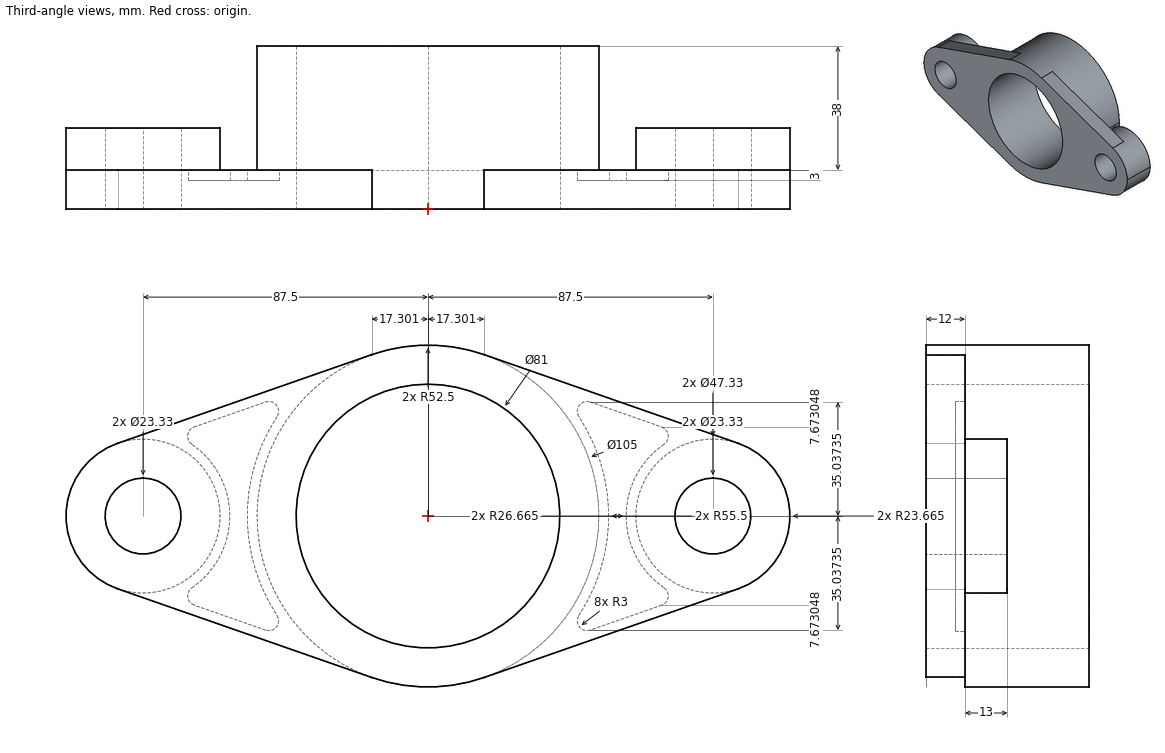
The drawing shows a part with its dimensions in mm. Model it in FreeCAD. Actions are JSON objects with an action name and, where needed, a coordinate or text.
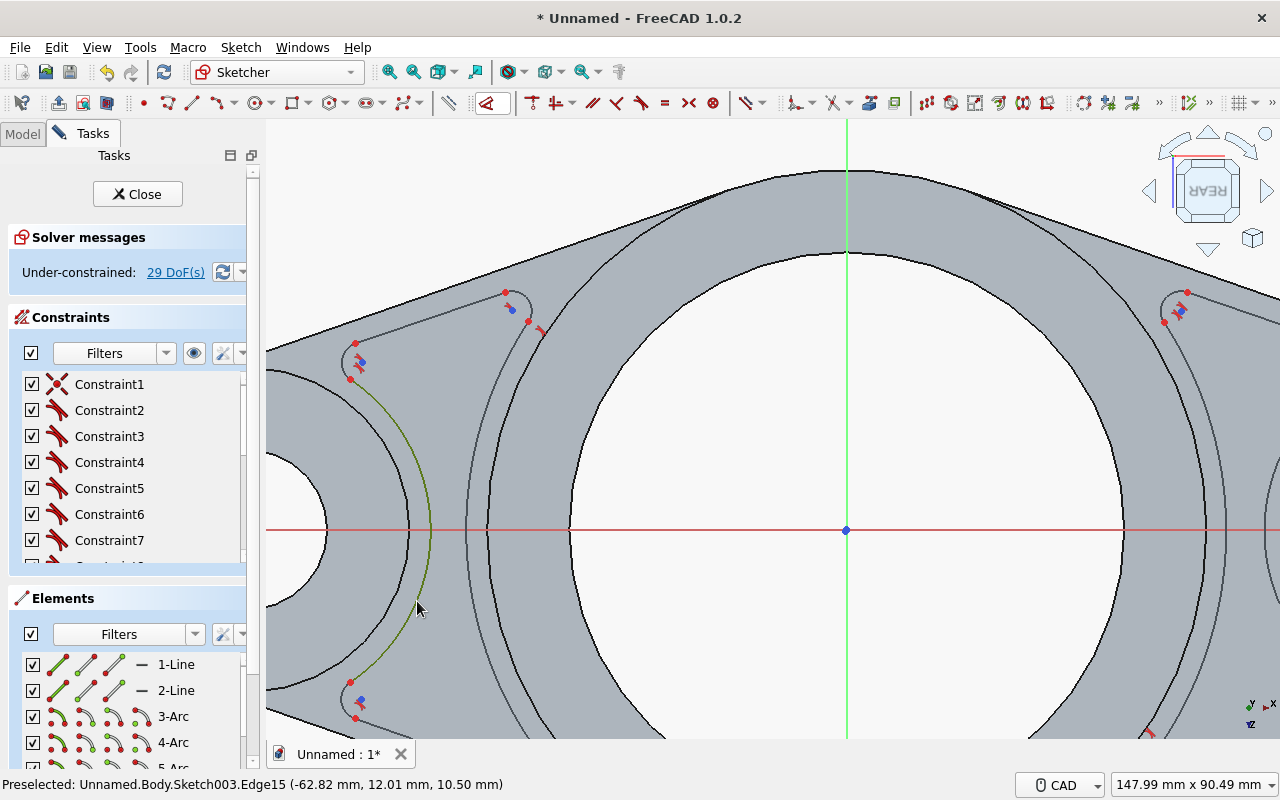
{"action": "left_click", "coordinate": [342, 693]}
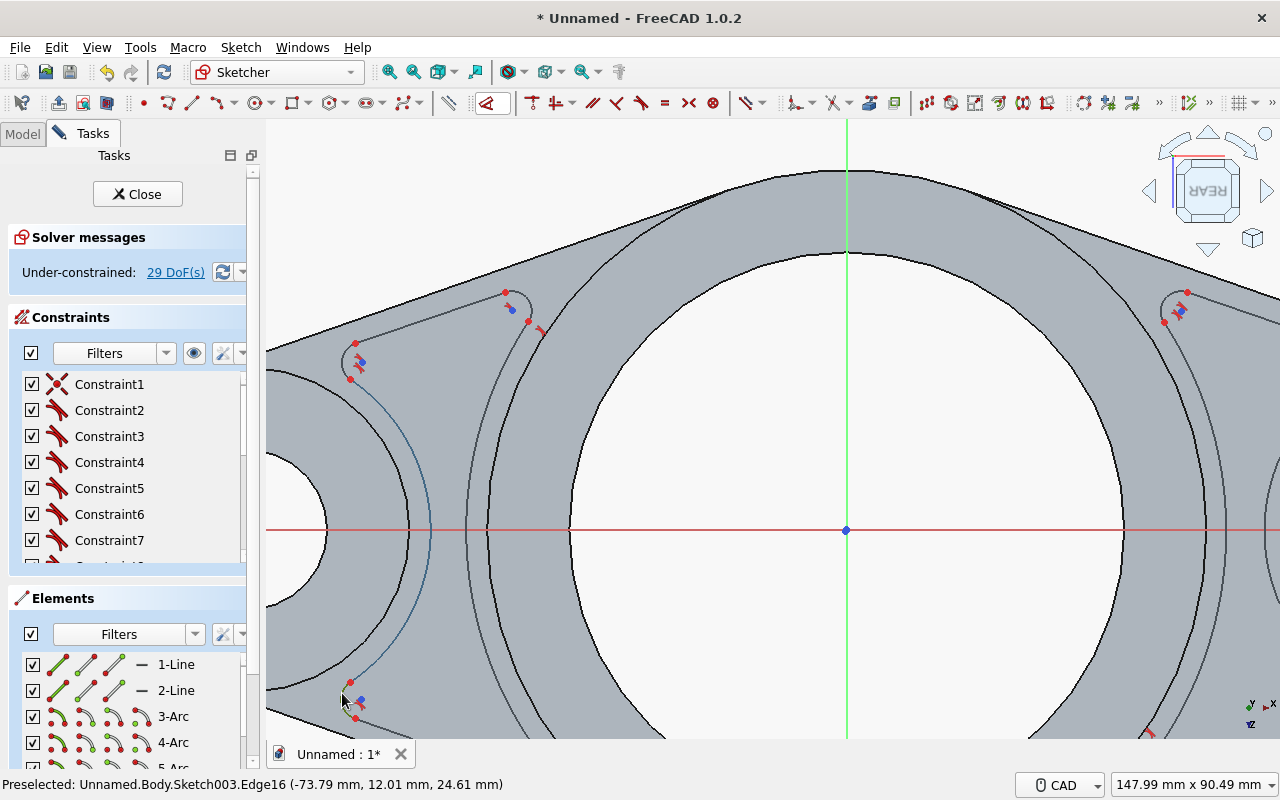
{"action": "left_click", "coordinate": [642, 104]}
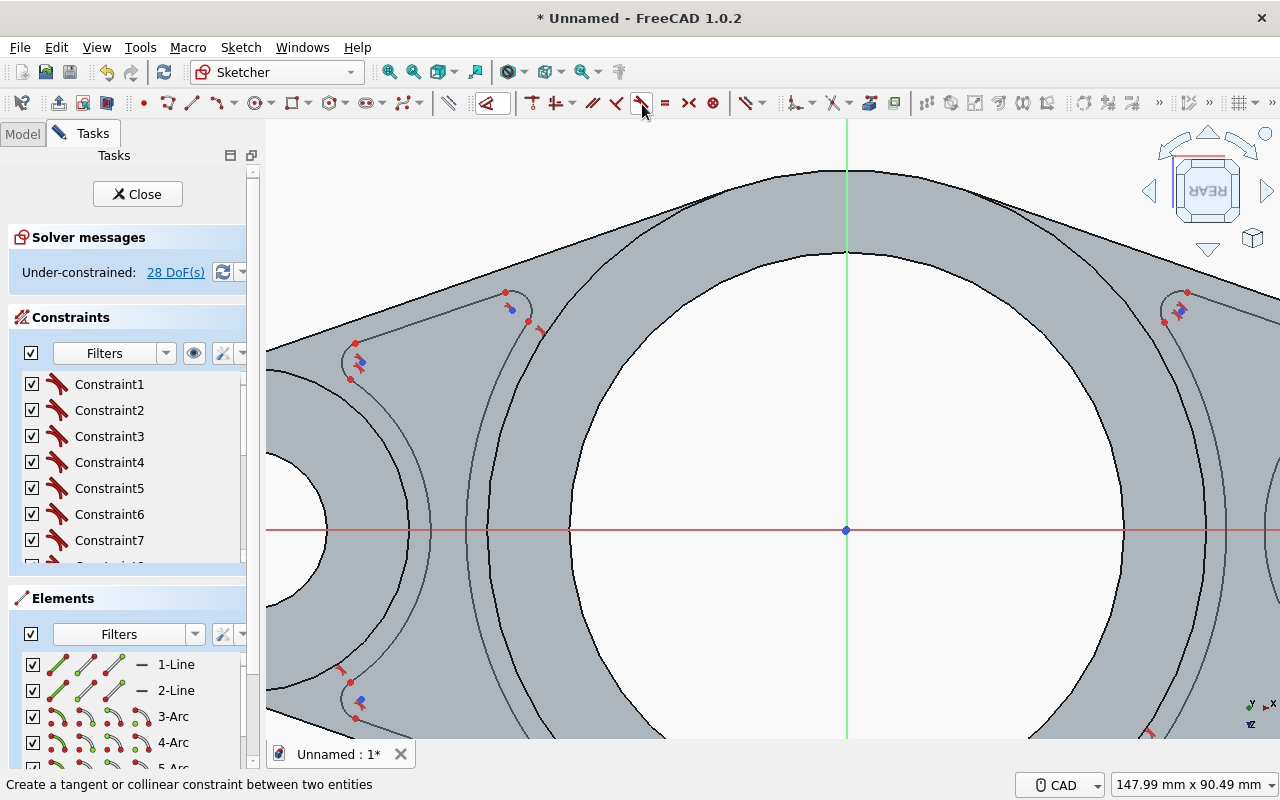
{"action": "scroll", "coordinate": [531, 306], "scroll_direction": "down", "scroll_amount": 3}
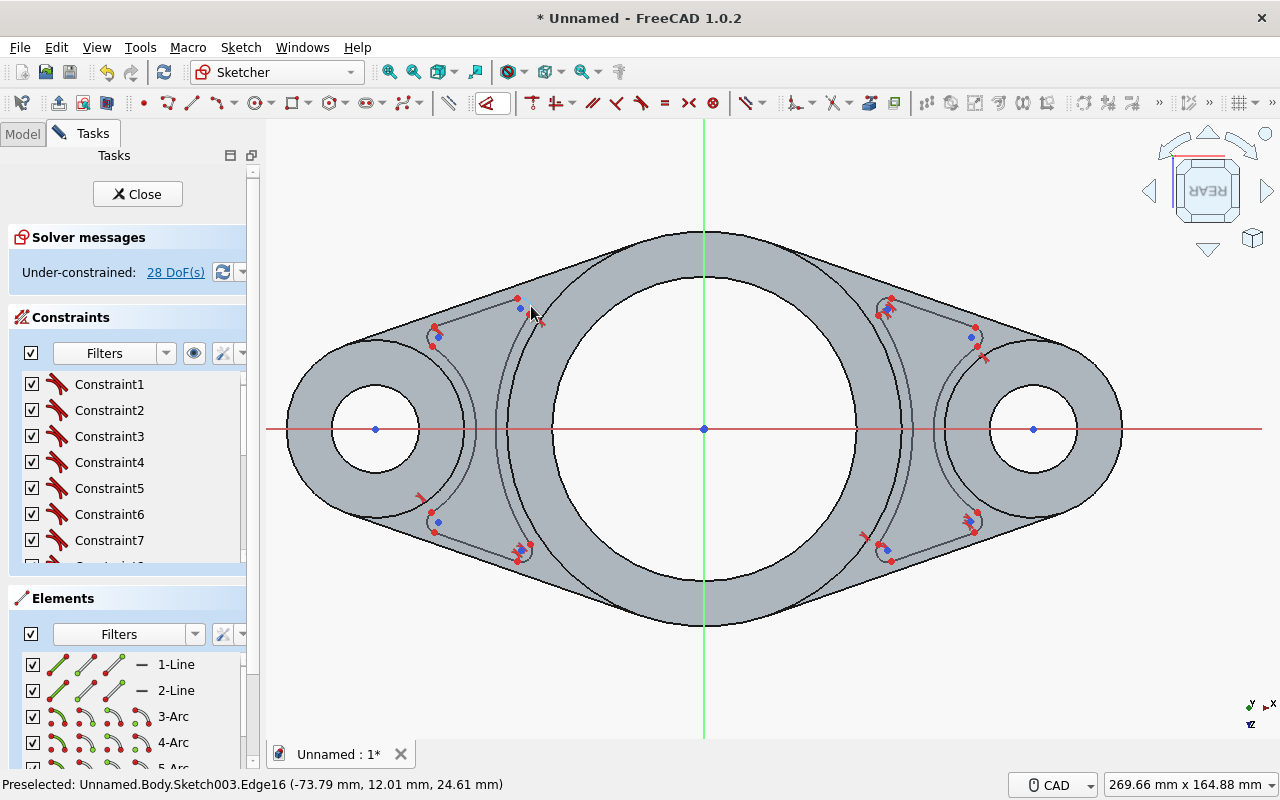
{"action": "left_click", "coordinate": [907, 478]}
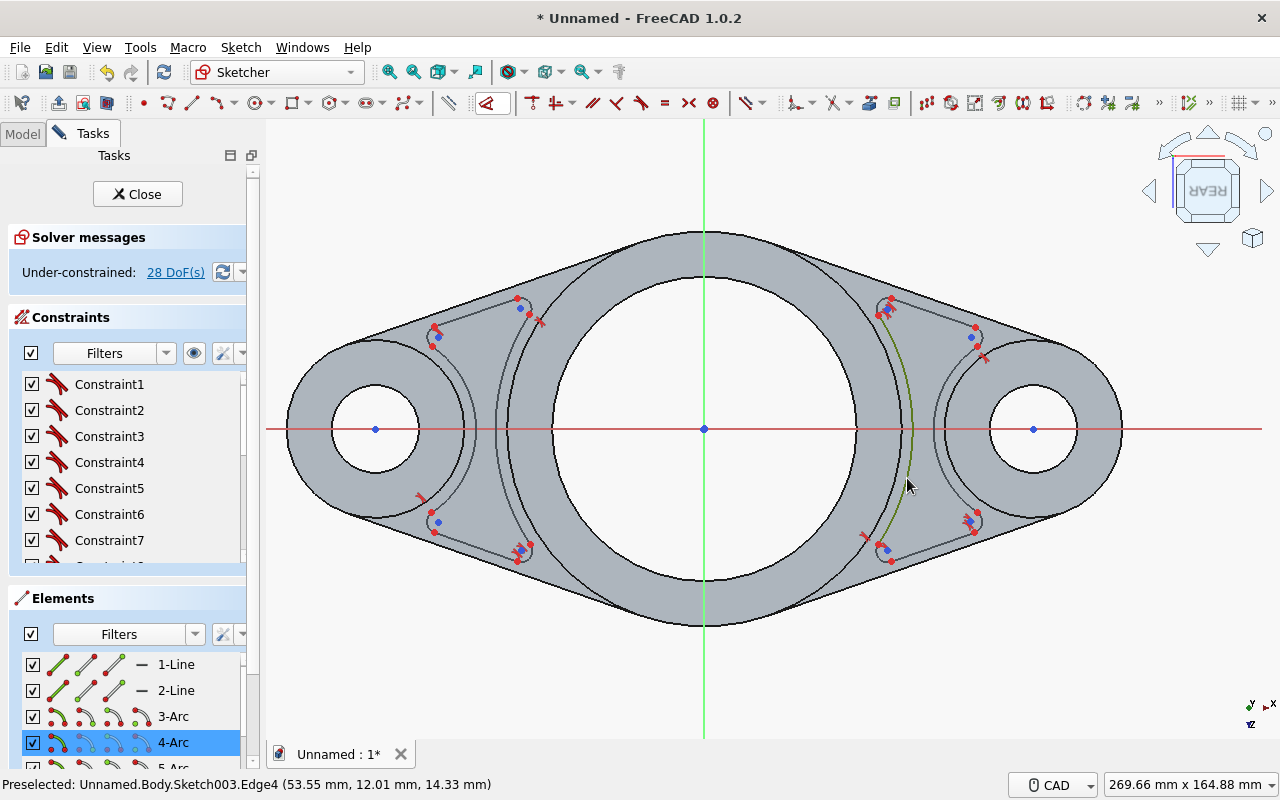
{"action": "left_click", "coordinate": [501, 381]}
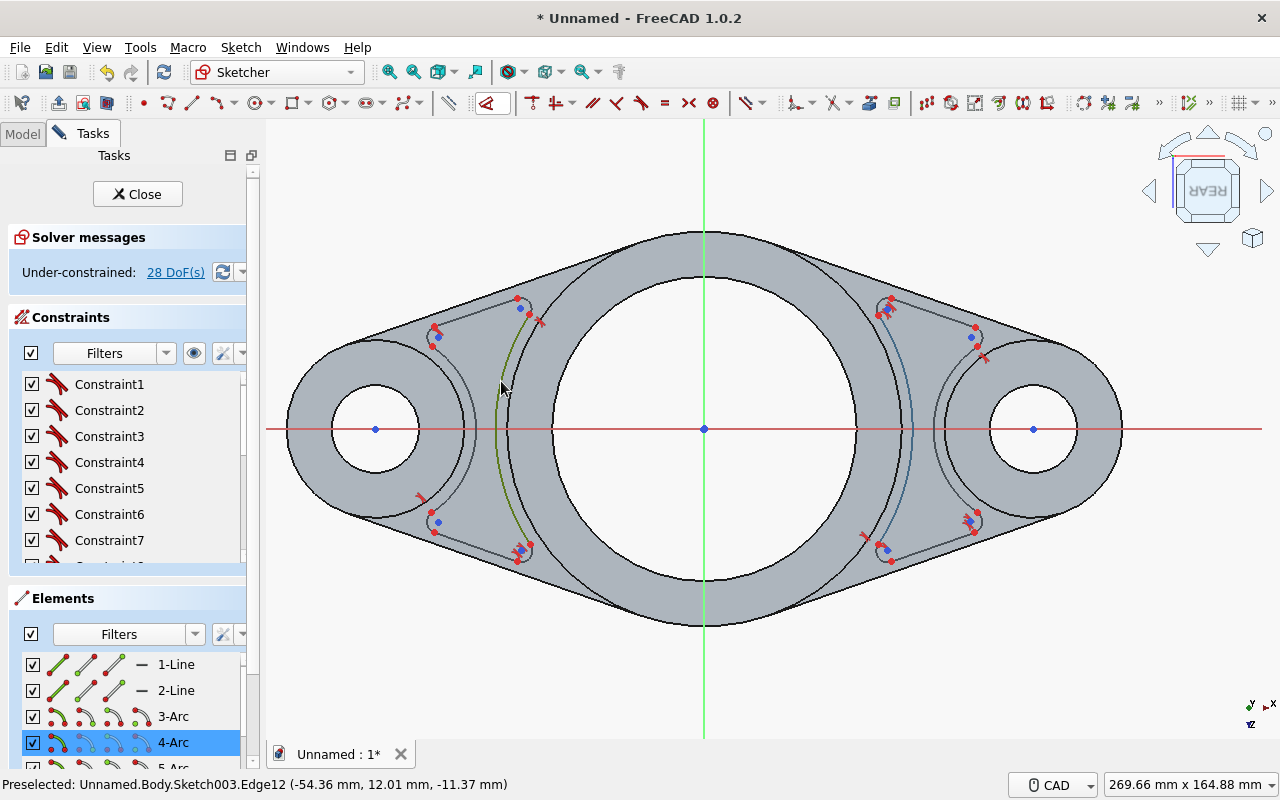
{"action": "left_click", "coordinate": [532, 104]}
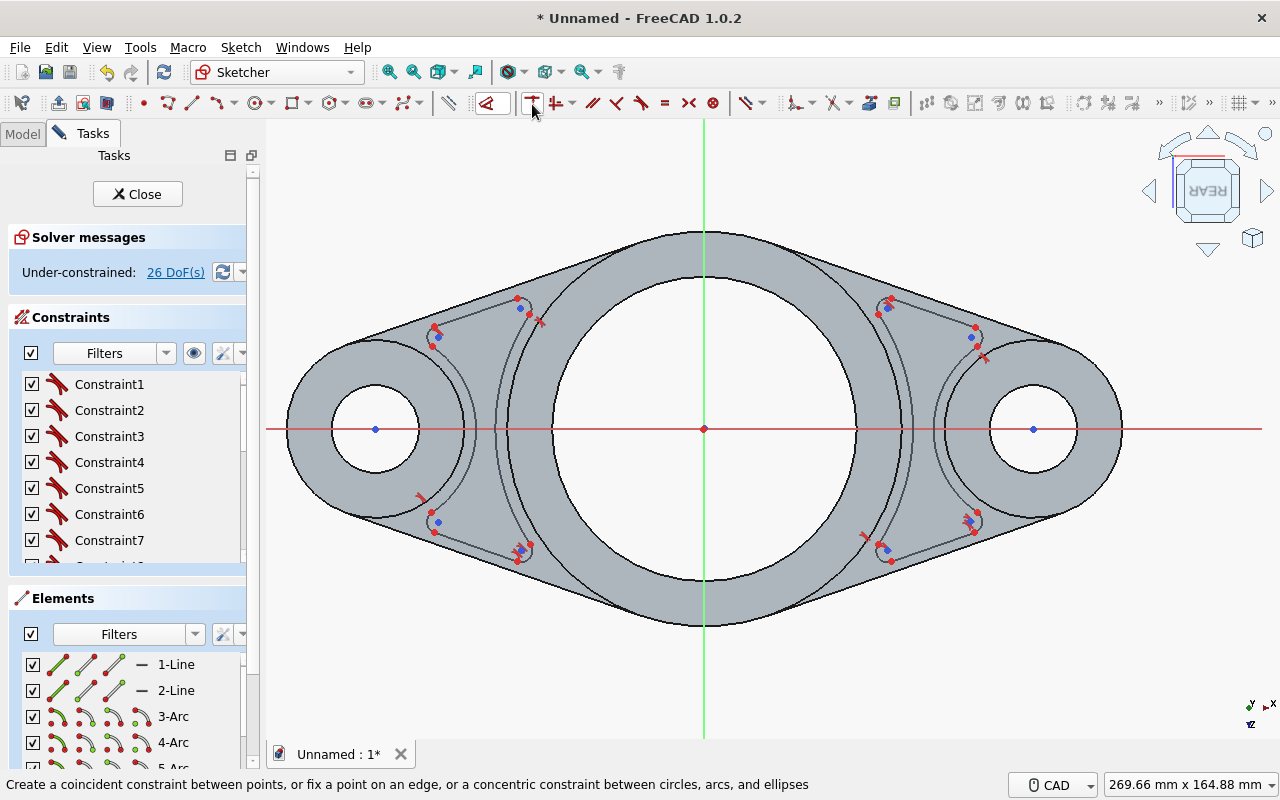
{"action": "scroll", "coordinate": [704, 429], "scroll_direction": "up", "scroll_amount": 7}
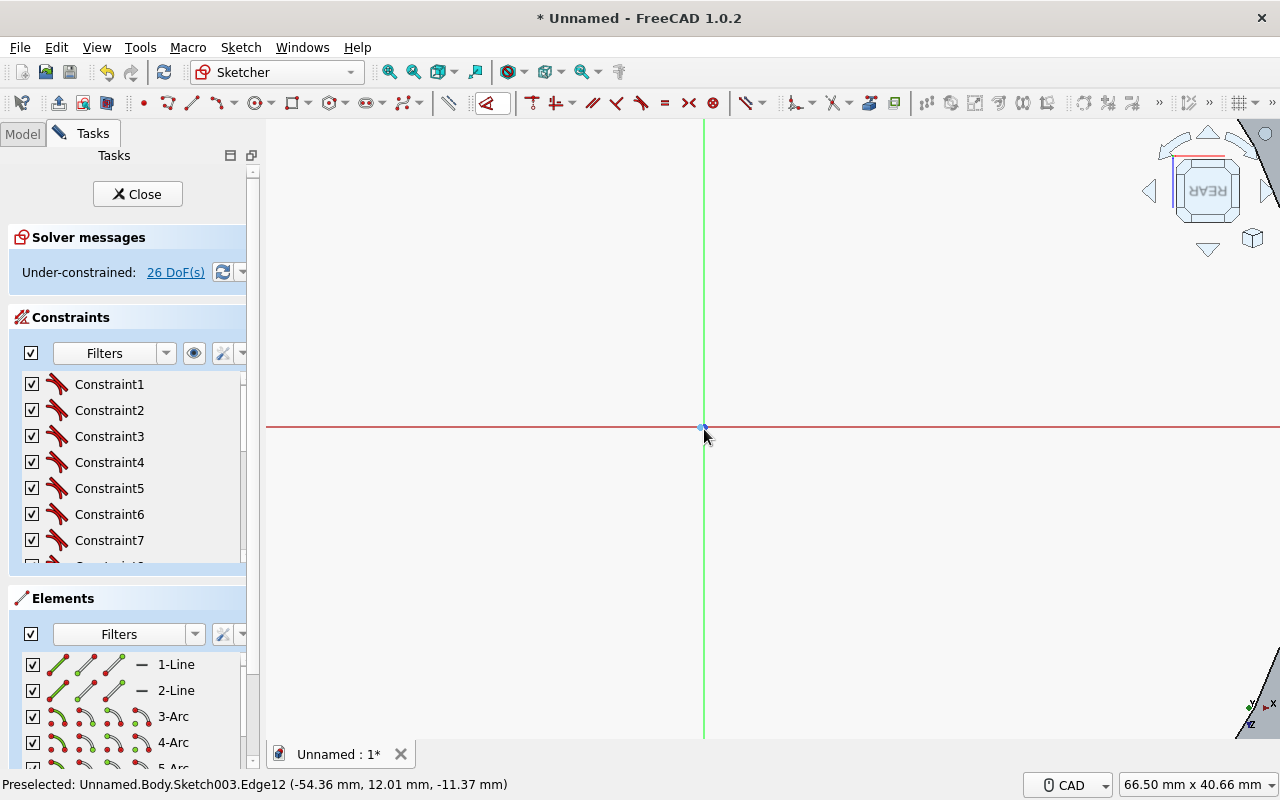
{"action": "left_click_drag", "start_coordinate": [691, 417], "coordinate": [714, 438]}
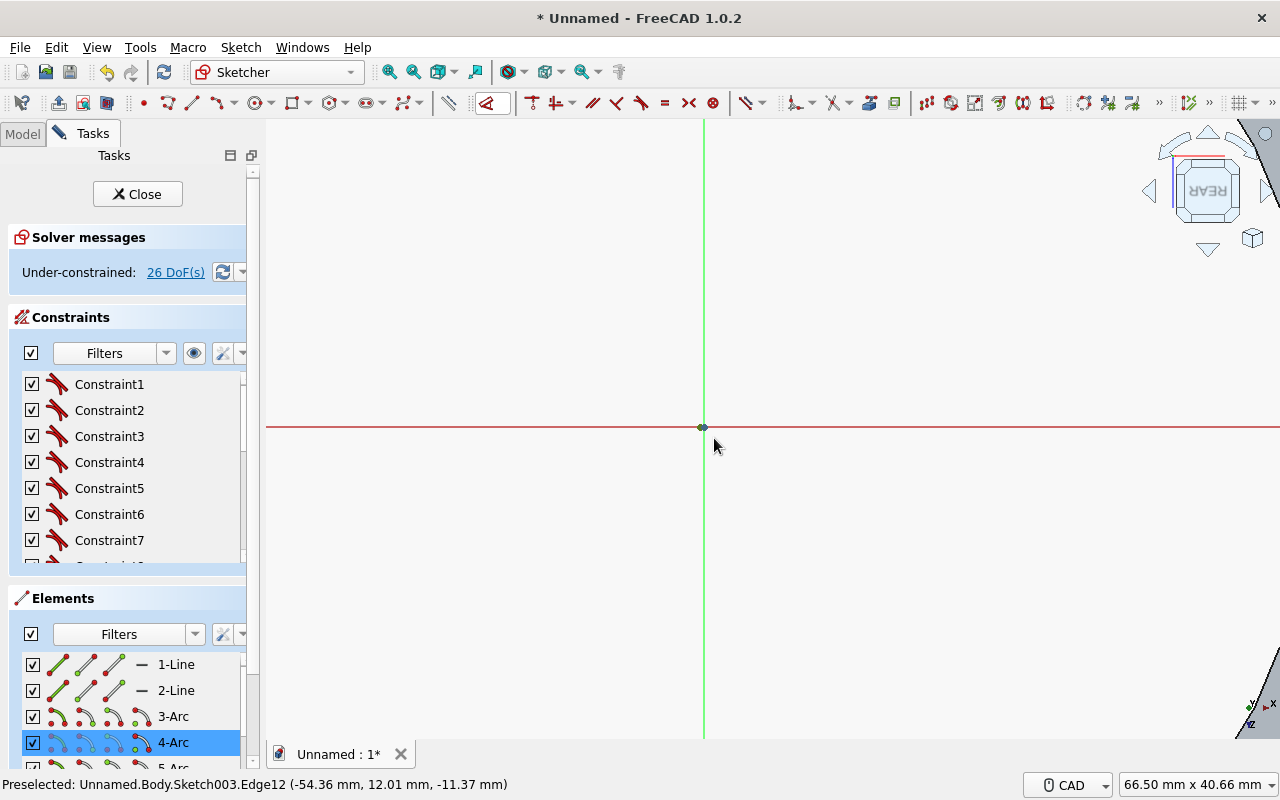
{"action": "left_click", "coordinate": [532, 104]}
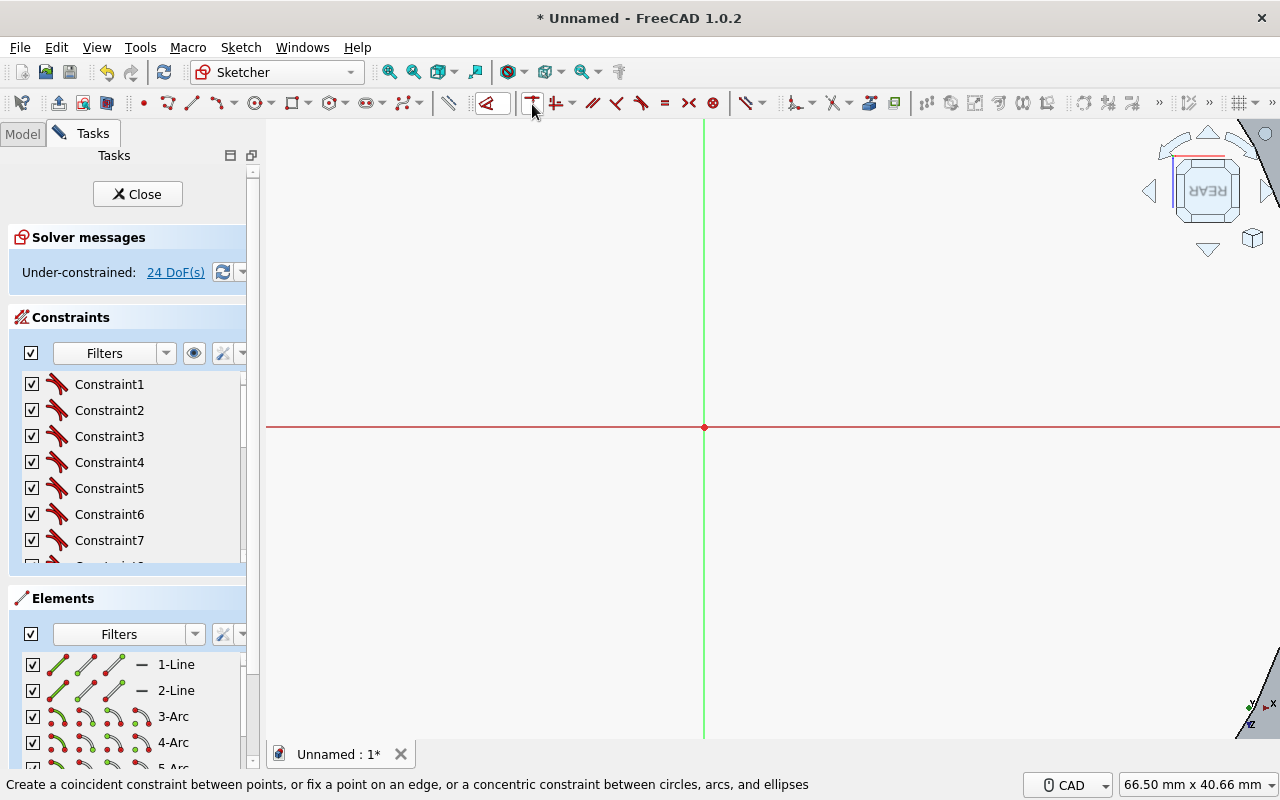
{"action": "scroll", "coordinate": [705, 430], "scroll_direction": "down", "scroll_amount": 7}